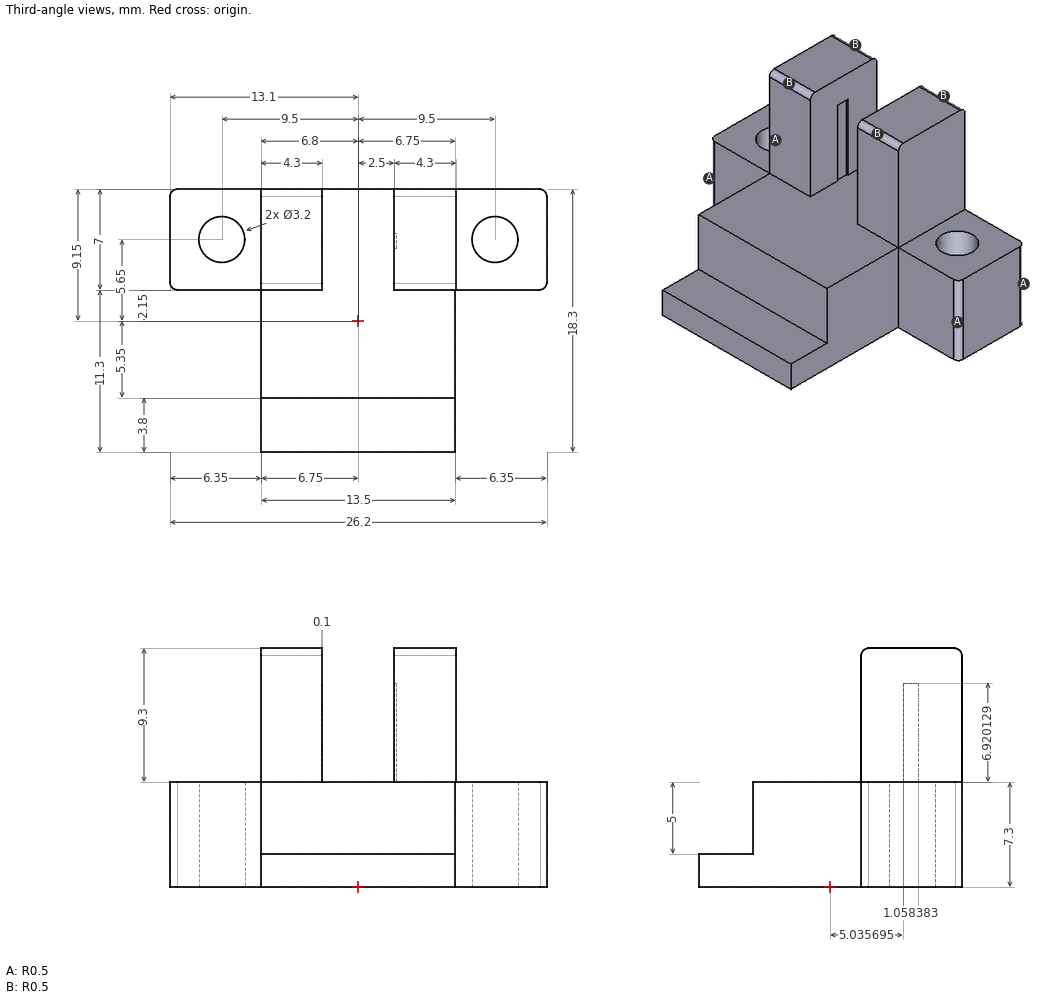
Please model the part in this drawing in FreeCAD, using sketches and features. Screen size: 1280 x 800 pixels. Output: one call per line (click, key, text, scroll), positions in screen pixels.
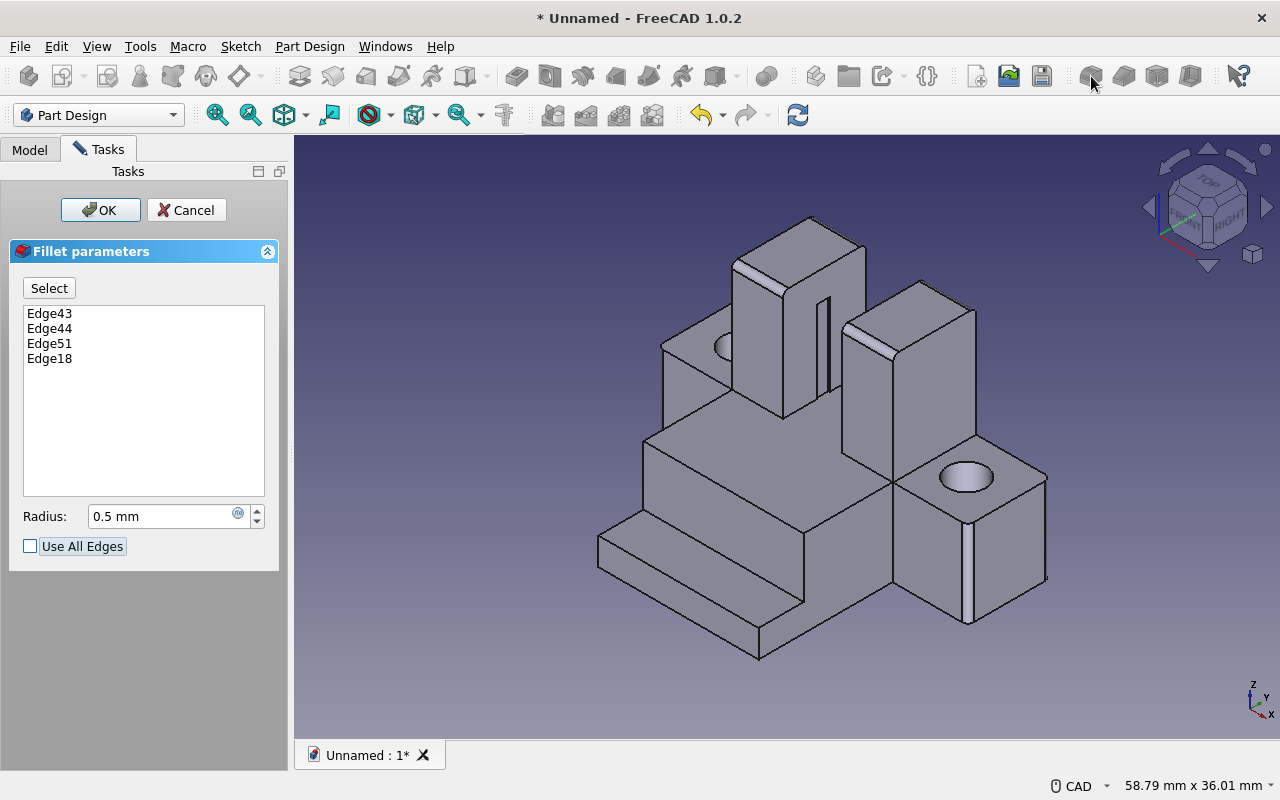
click(101, 210)